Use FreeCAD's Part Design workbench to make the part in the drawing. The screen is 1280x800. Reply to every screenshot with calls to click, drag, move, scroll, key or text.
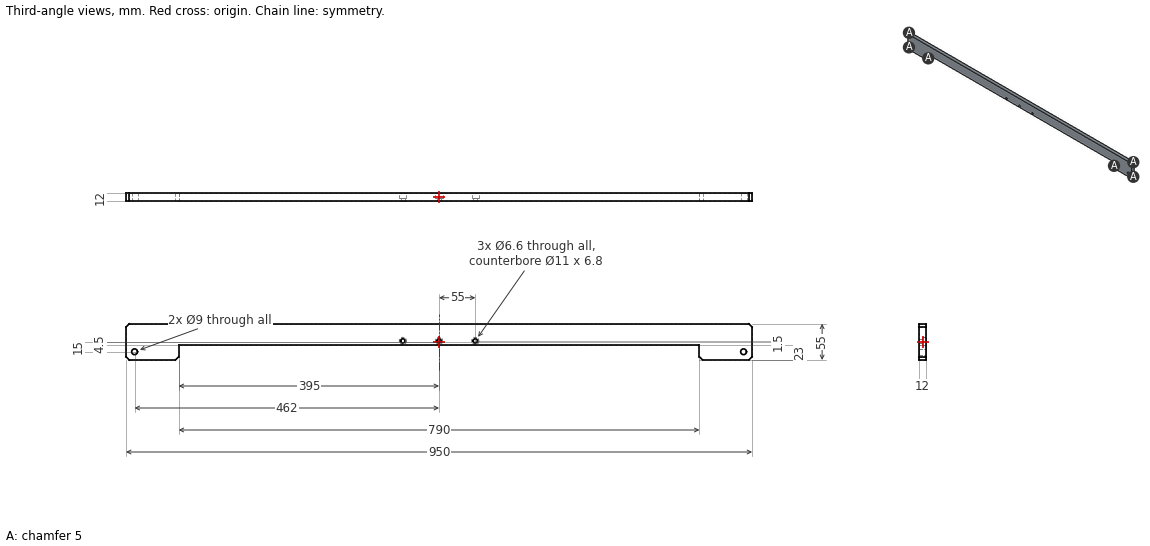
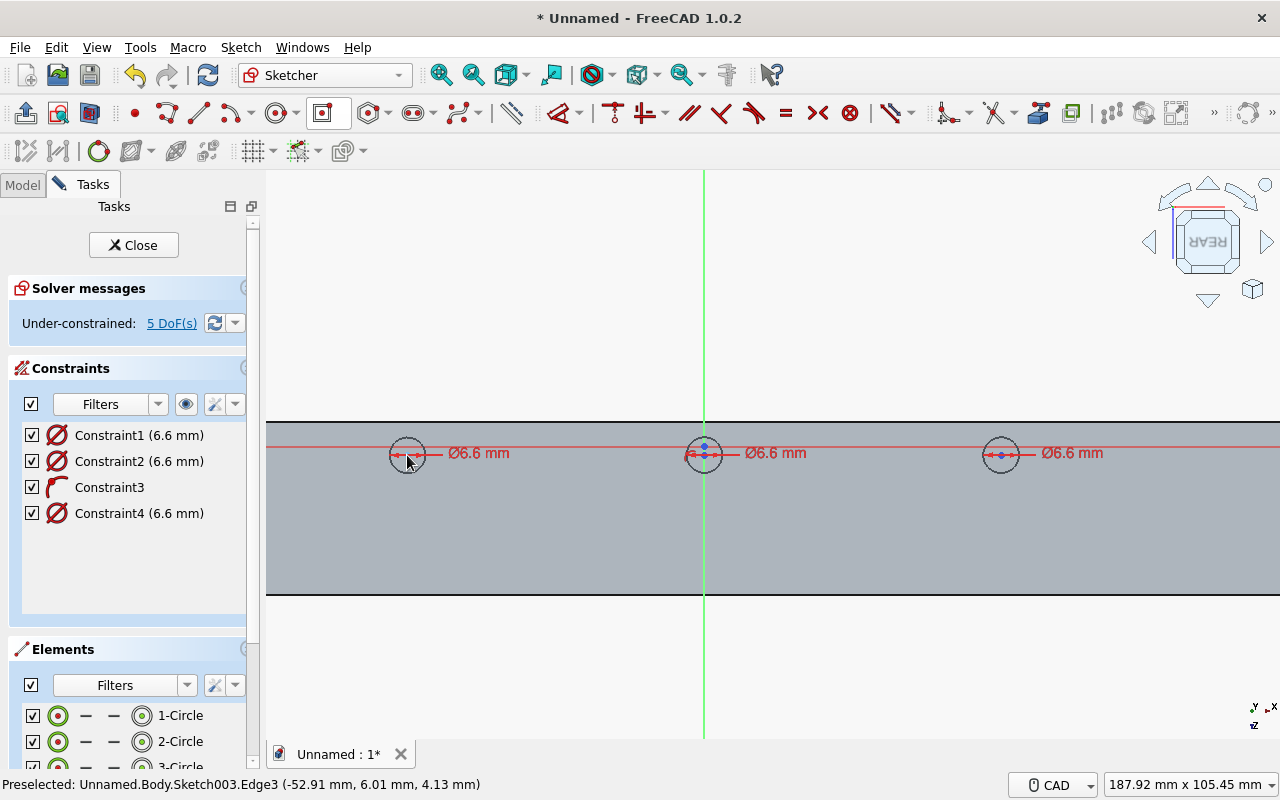
click(1001, 455)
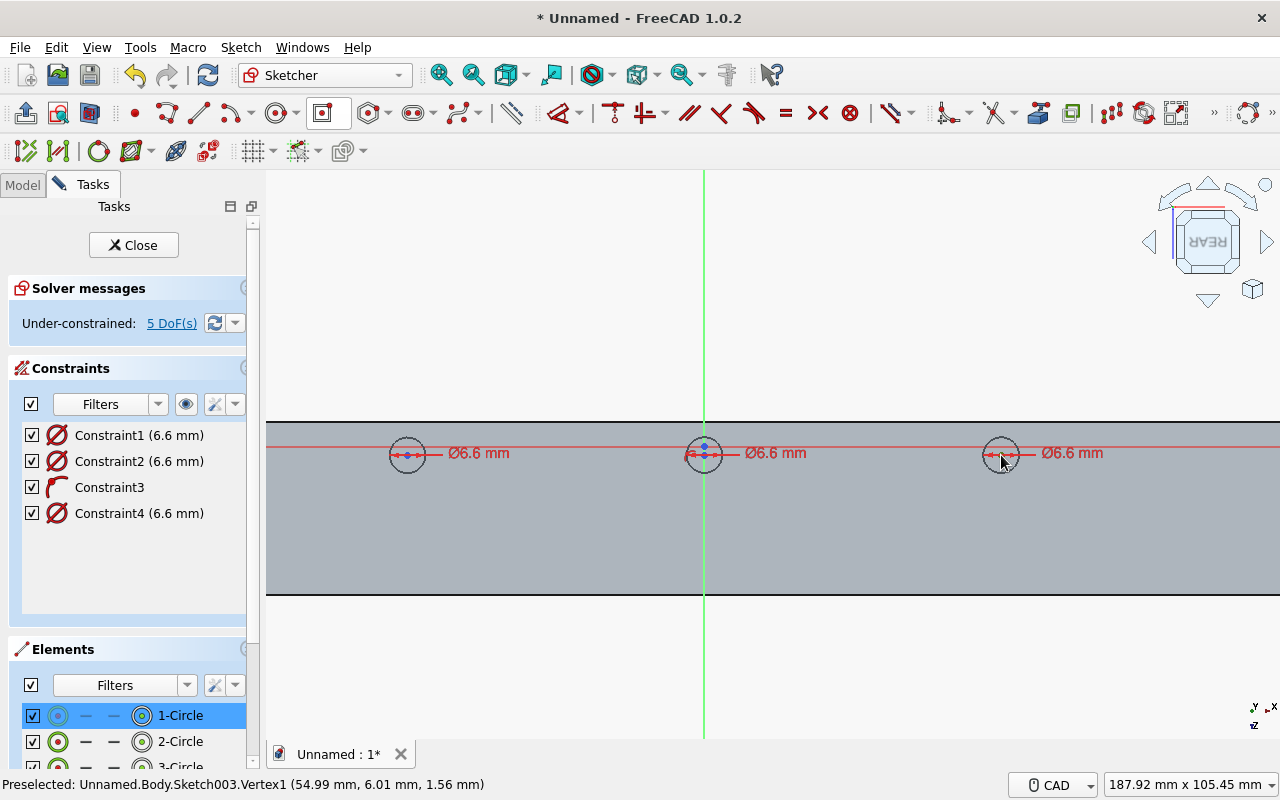
click(408, 455)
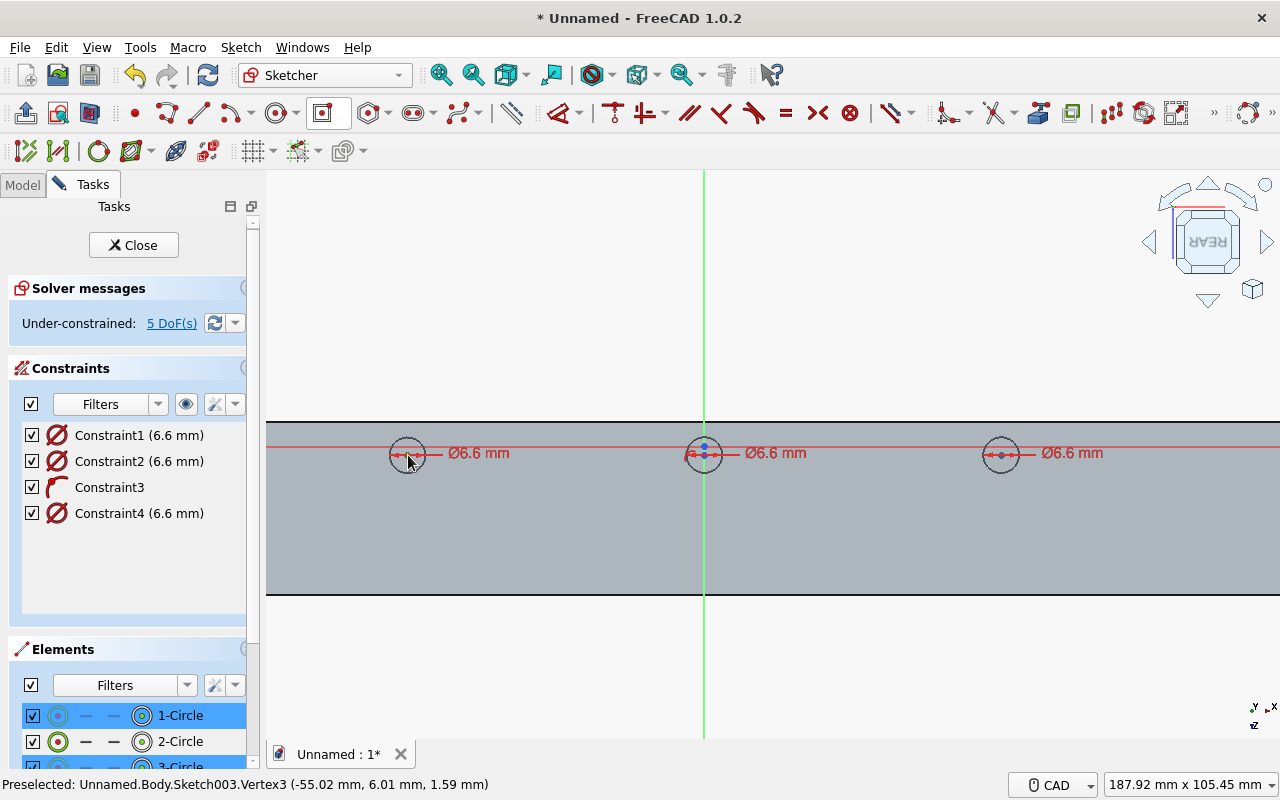
click(704, 674)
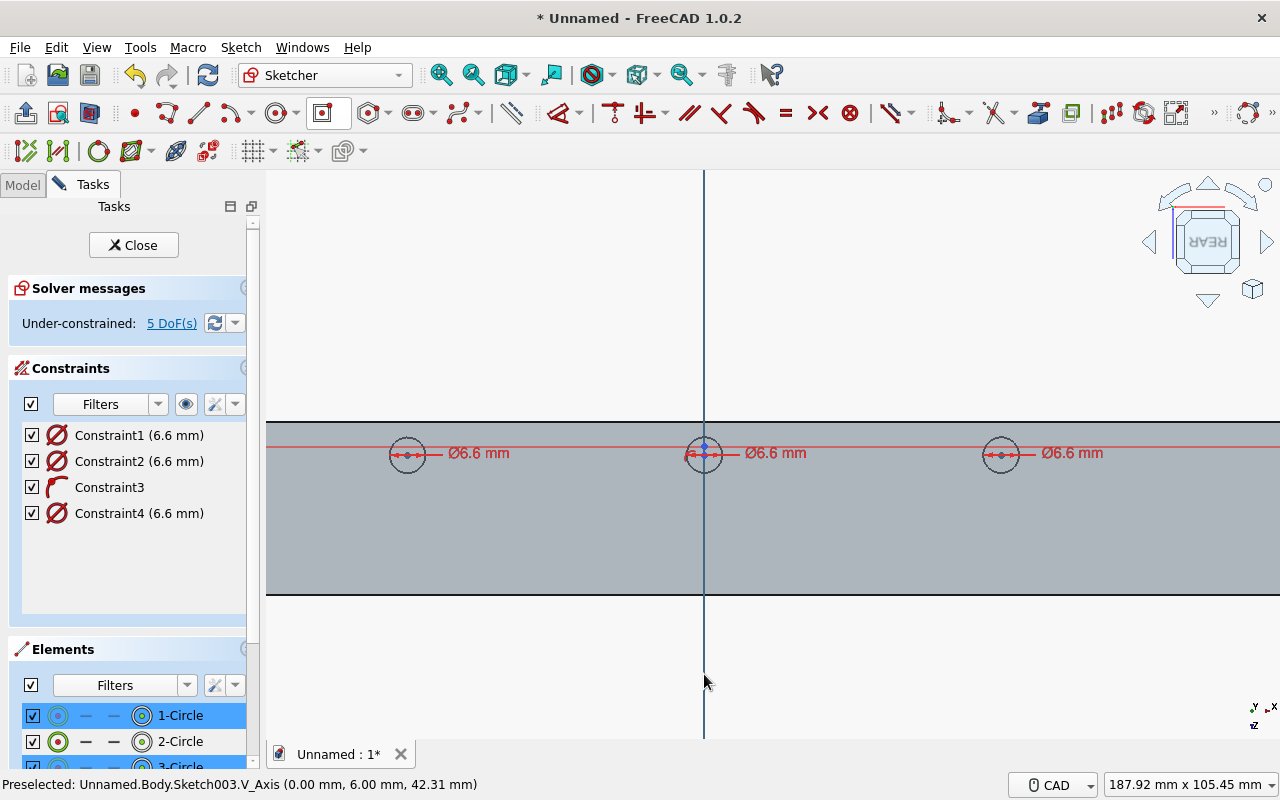
click(818, 114)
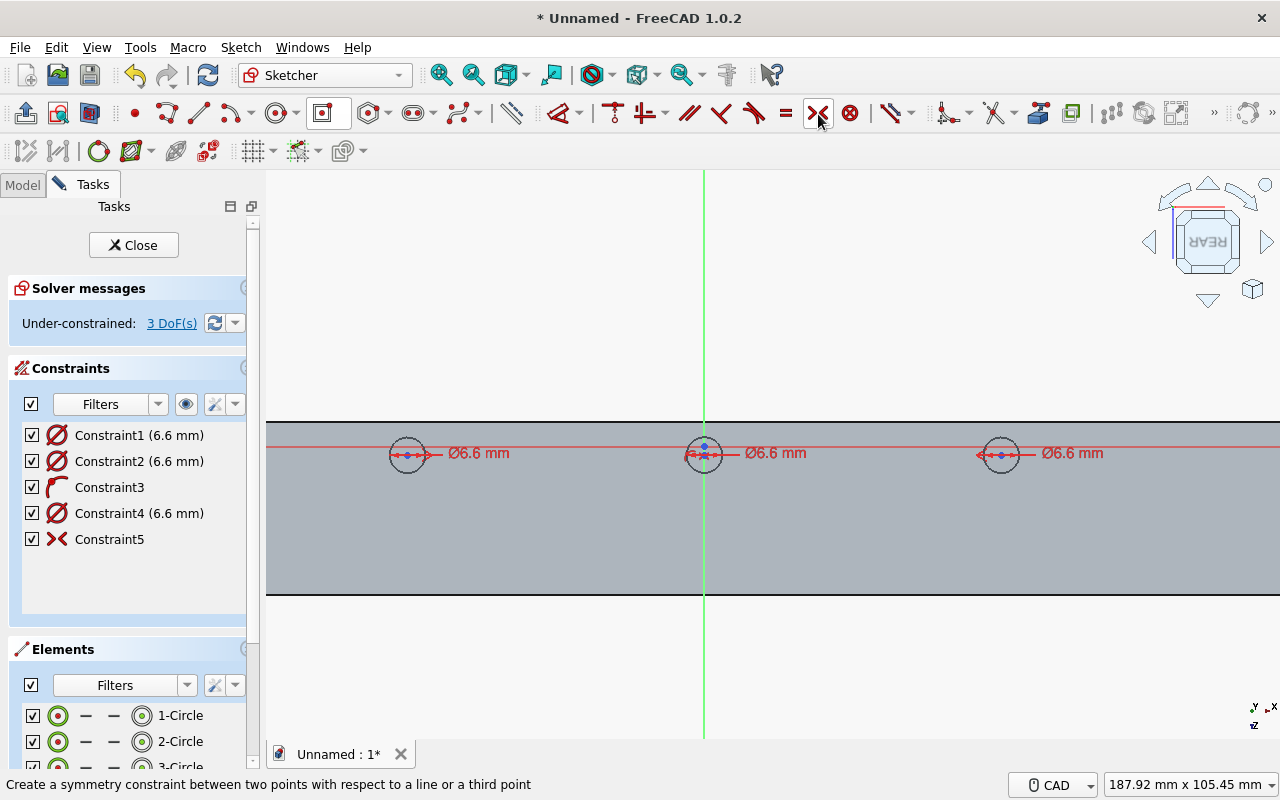
click(558, 114)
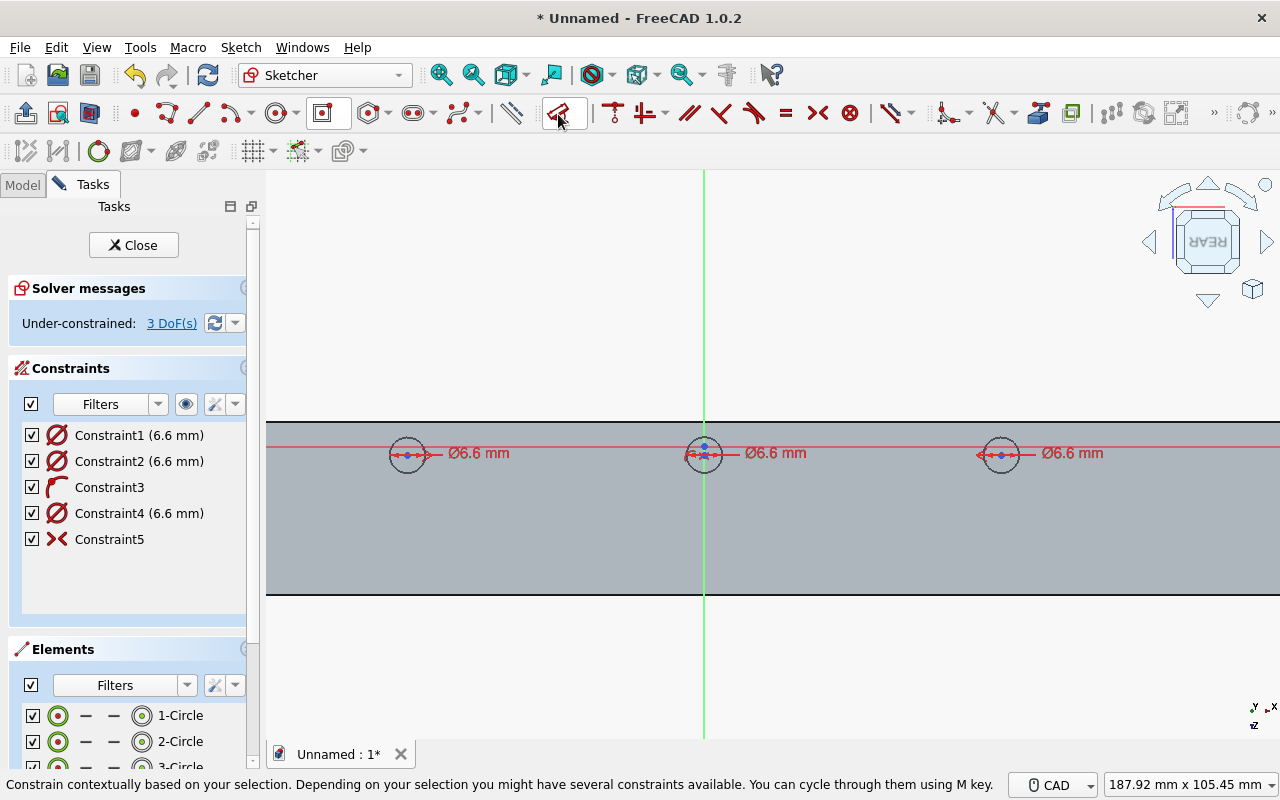
click(1001, 455)
click(853, 413)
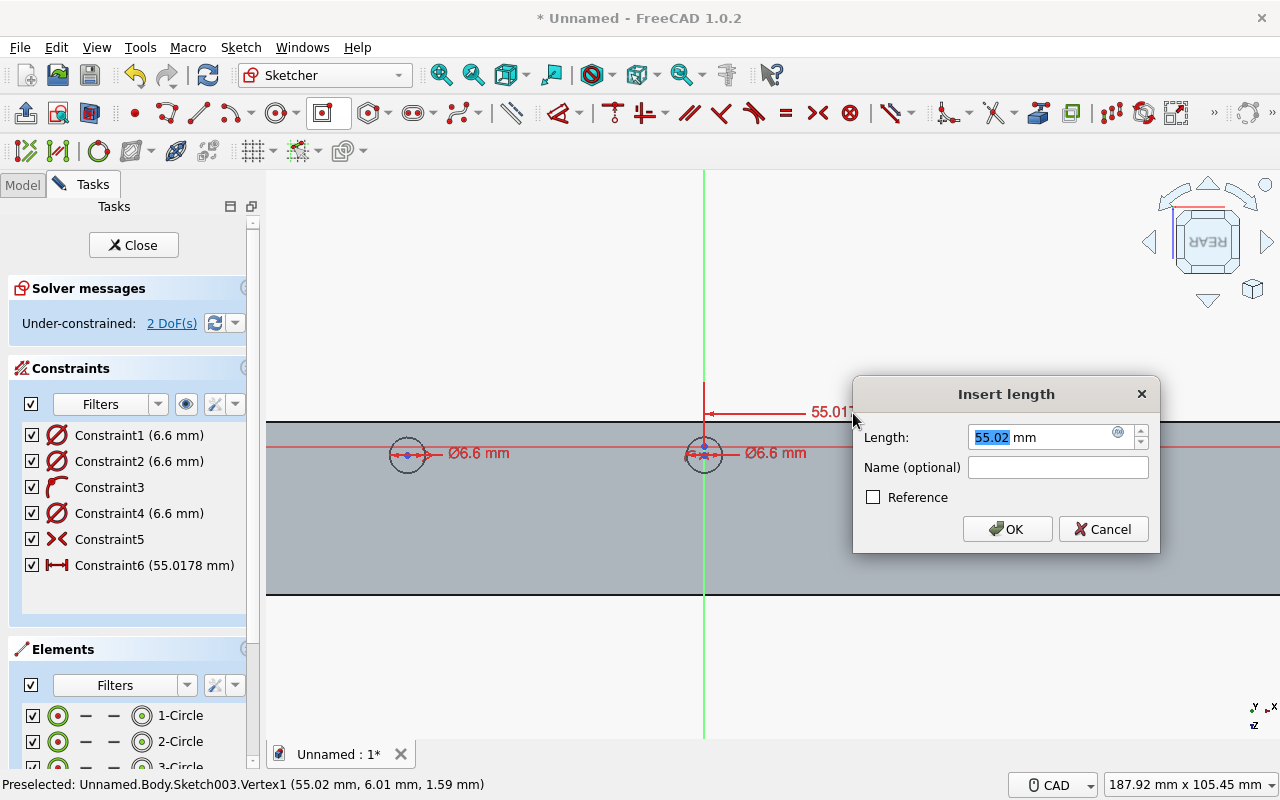
text(55)
key(Return)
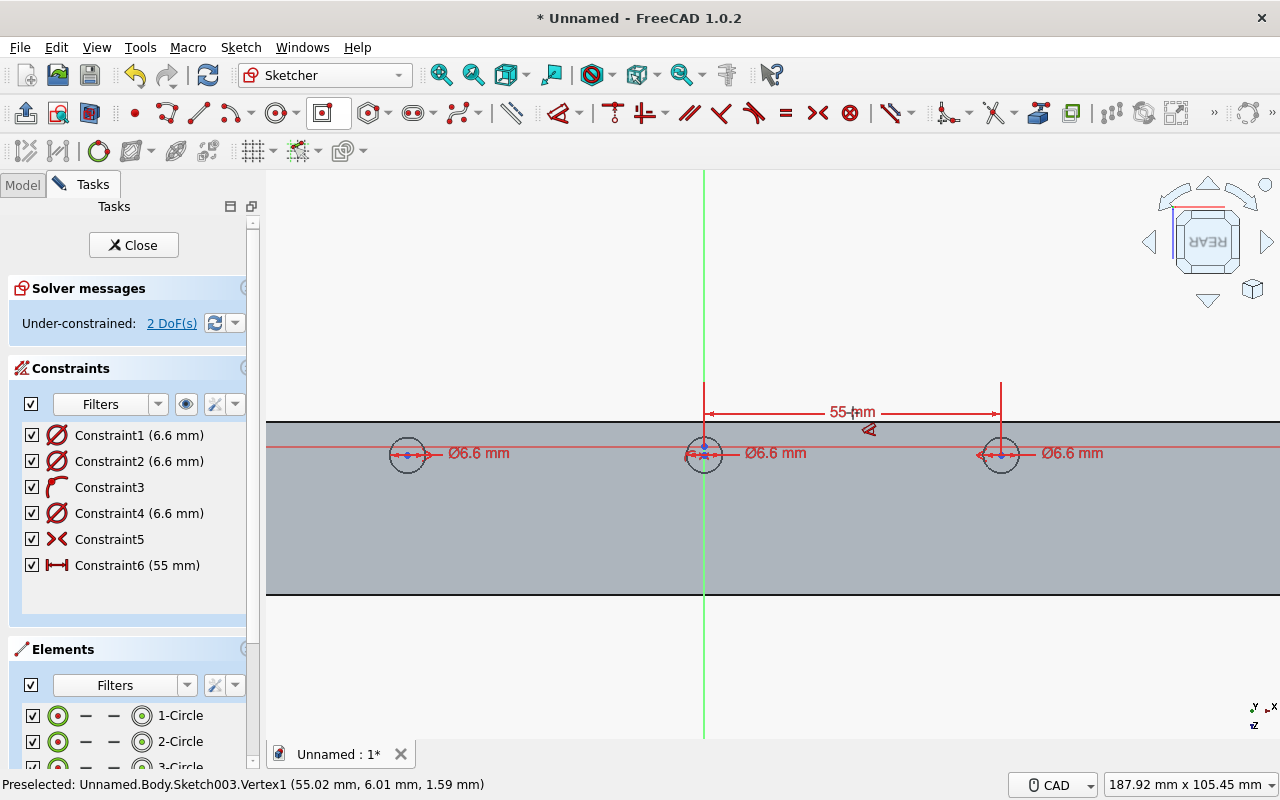
scroll(1001, 455, up, 8)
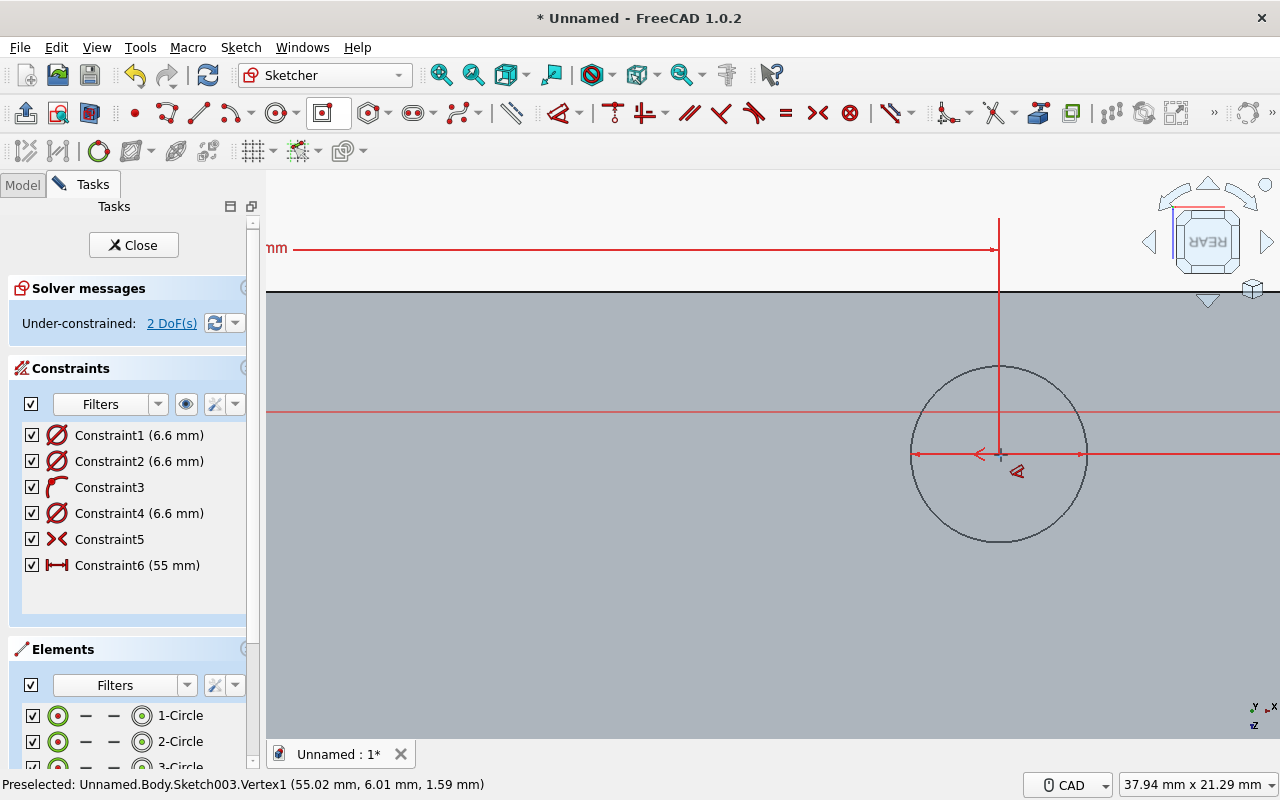
click(999, 454)
click(1033, 433)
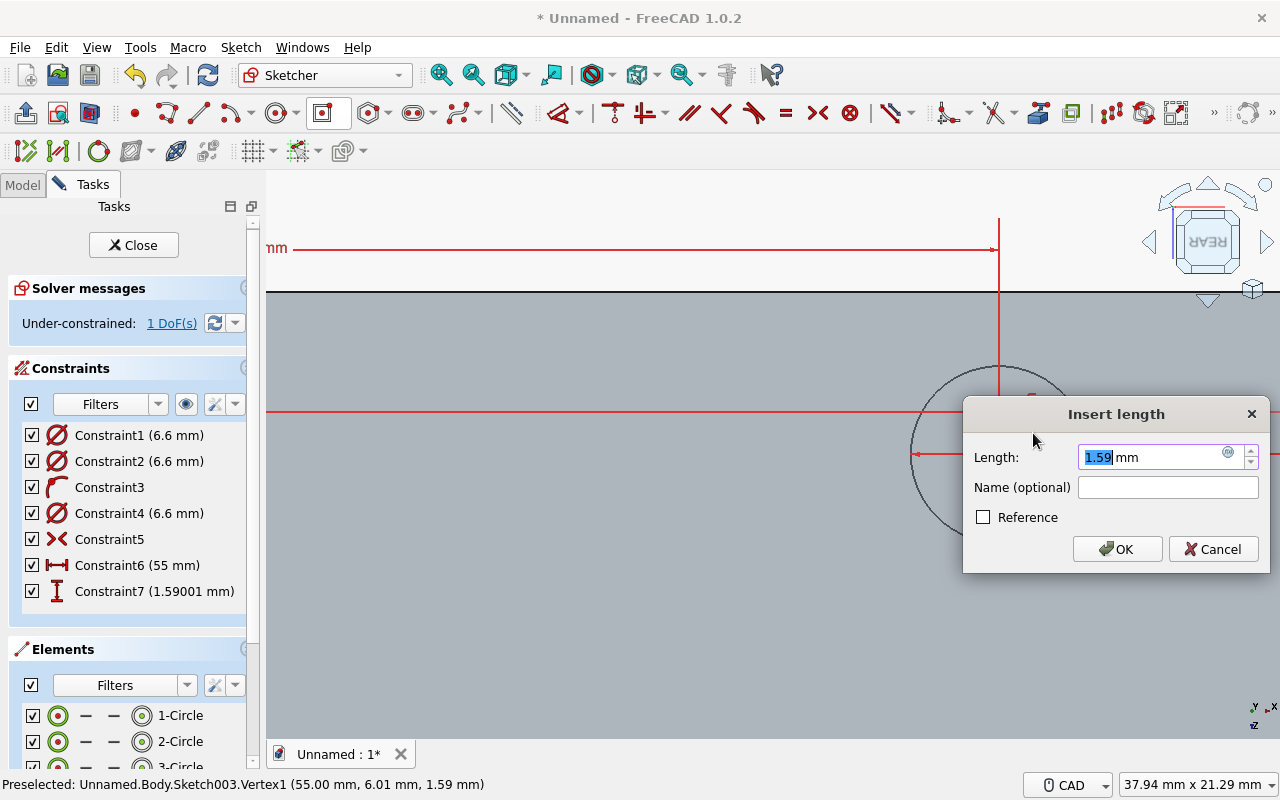
text(1.5)
key(Return)